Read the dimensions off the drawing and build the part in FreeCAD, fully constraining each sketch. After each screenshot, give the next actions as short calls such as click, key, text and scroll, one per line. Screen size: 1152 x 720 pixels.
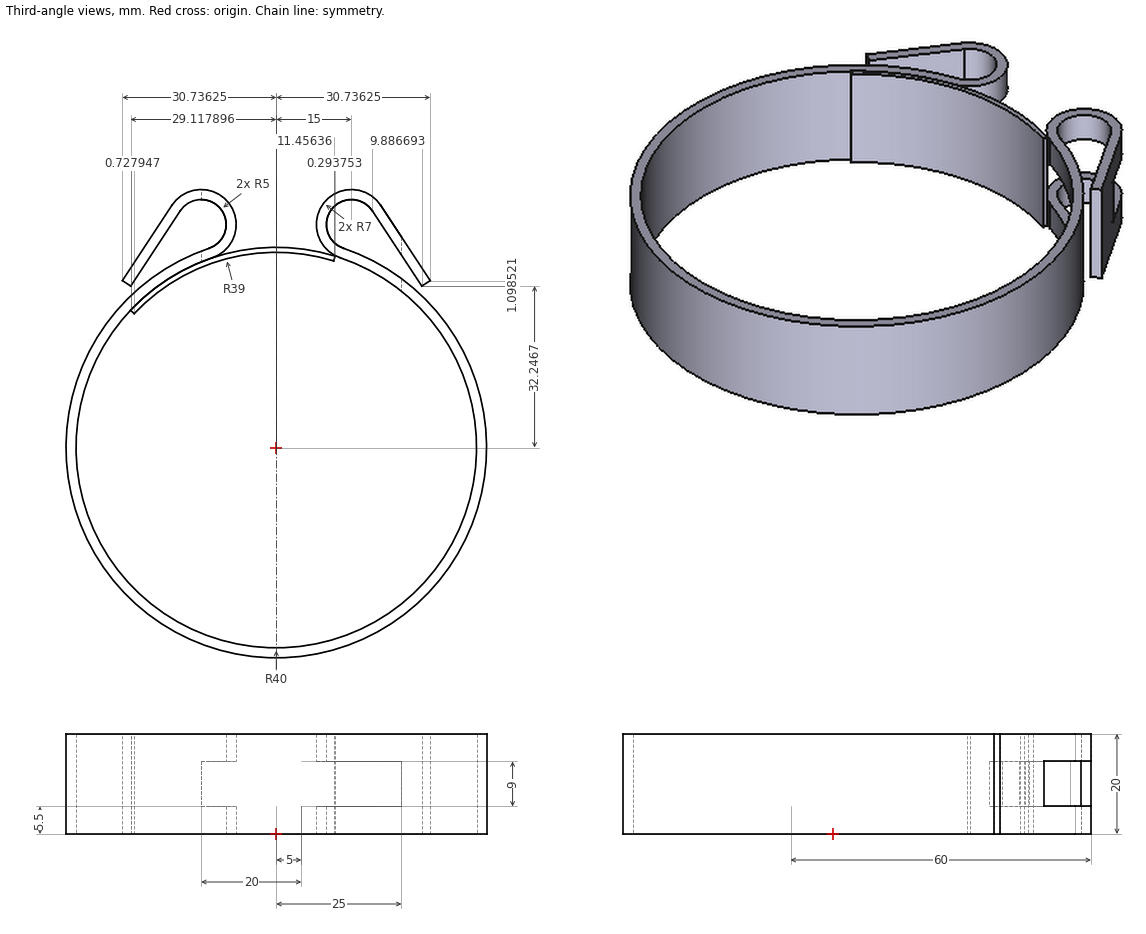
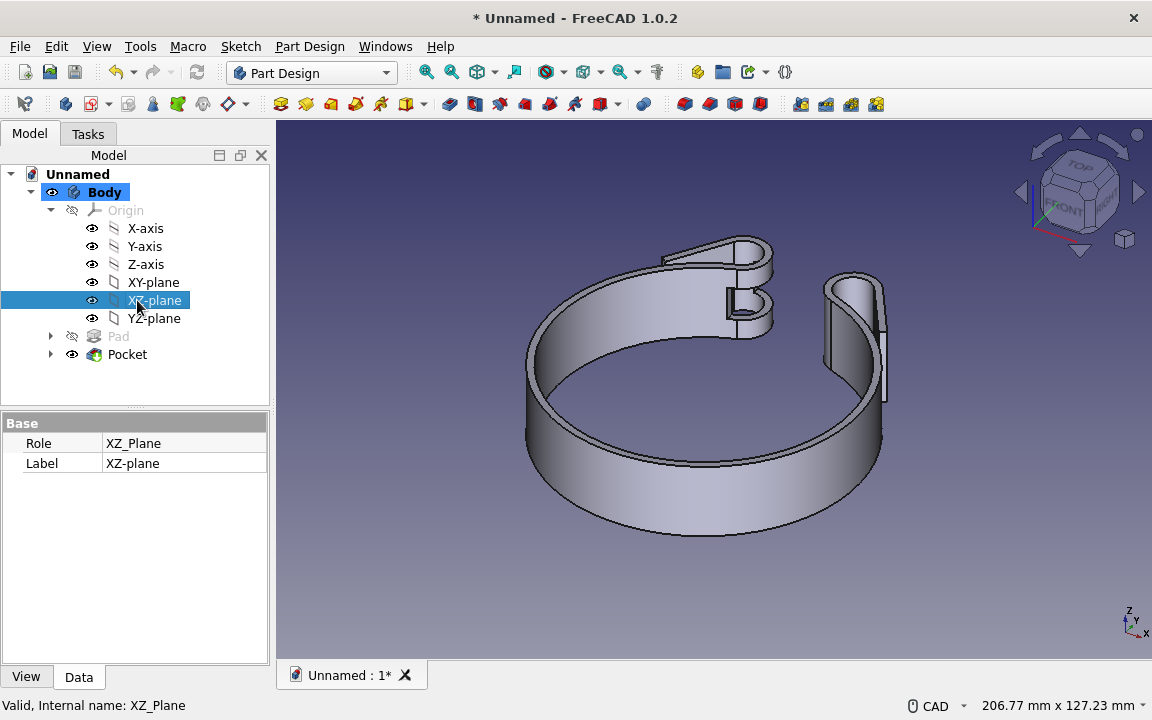
click(228, 104)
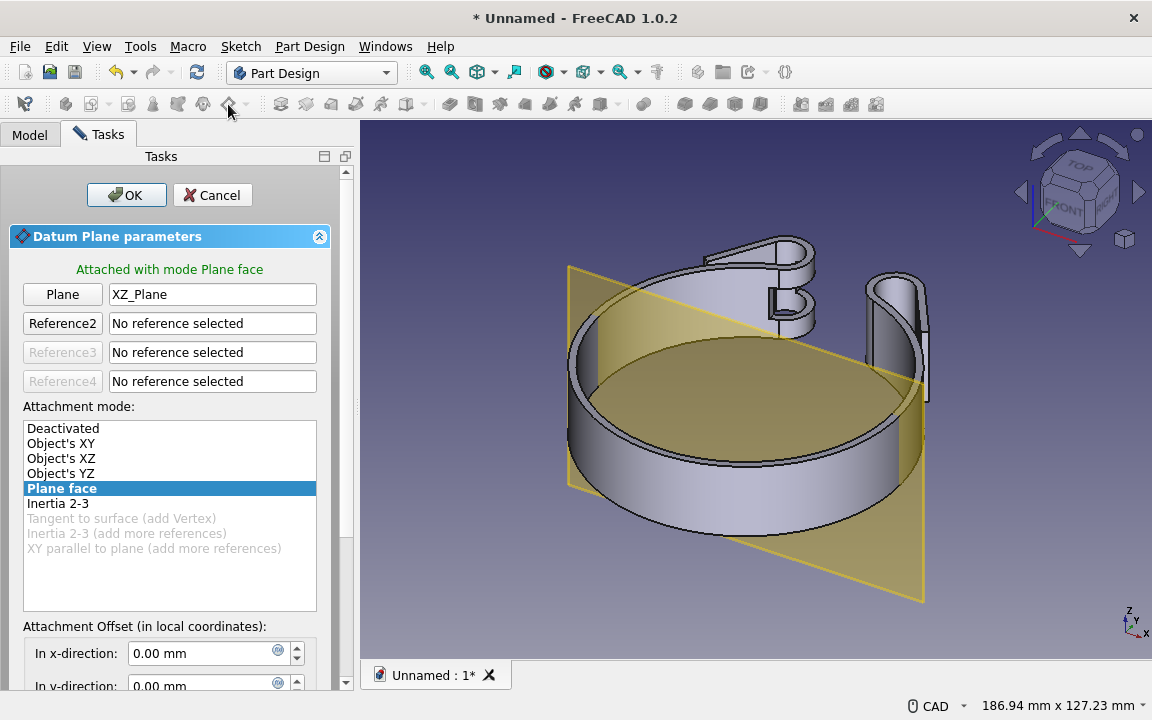
scroll(346, 428, down, 2)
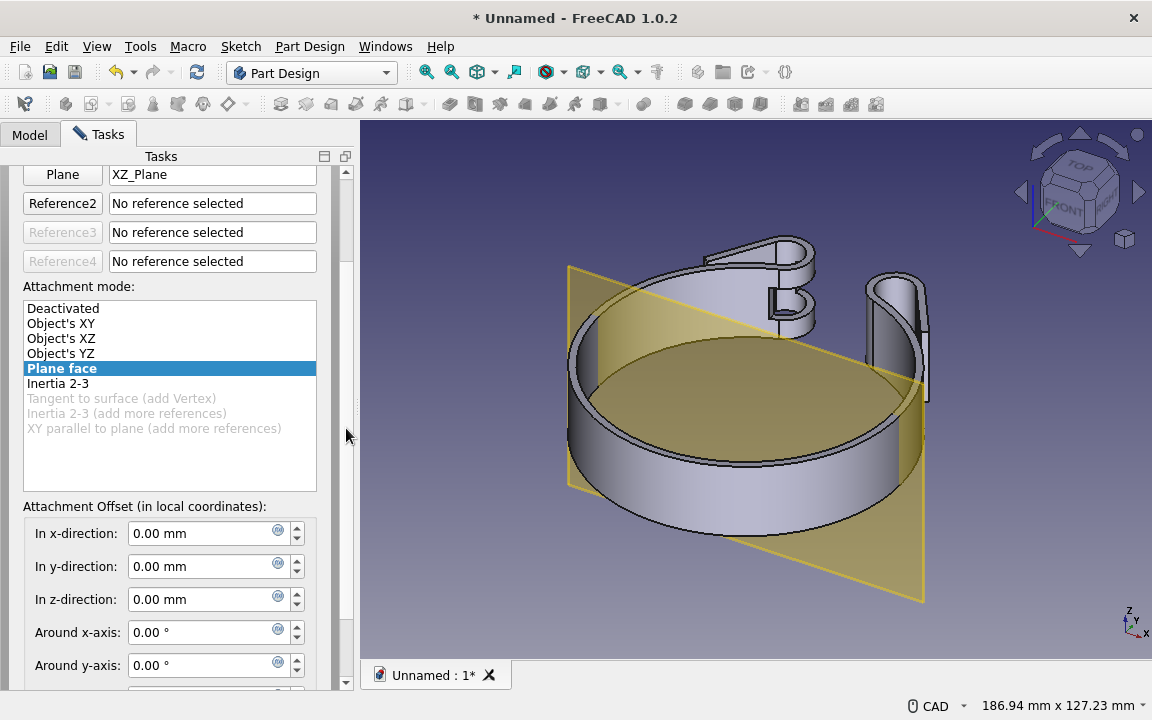
triple_click(210, 600)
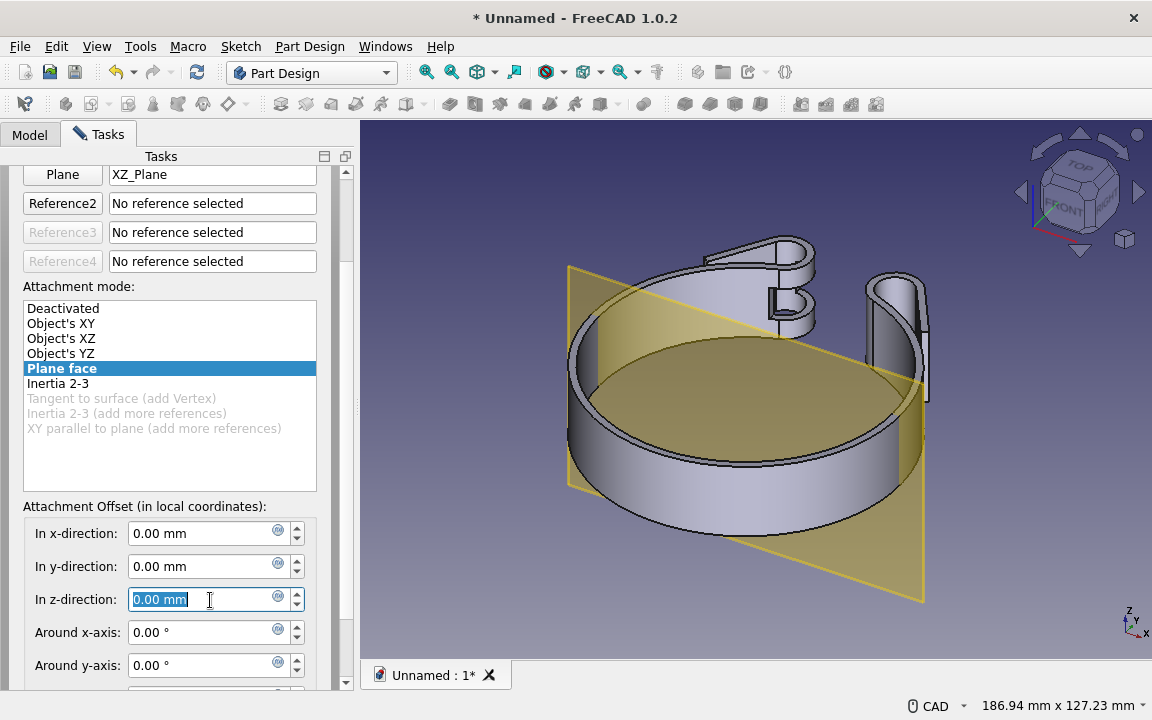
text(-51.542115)
key(Tab)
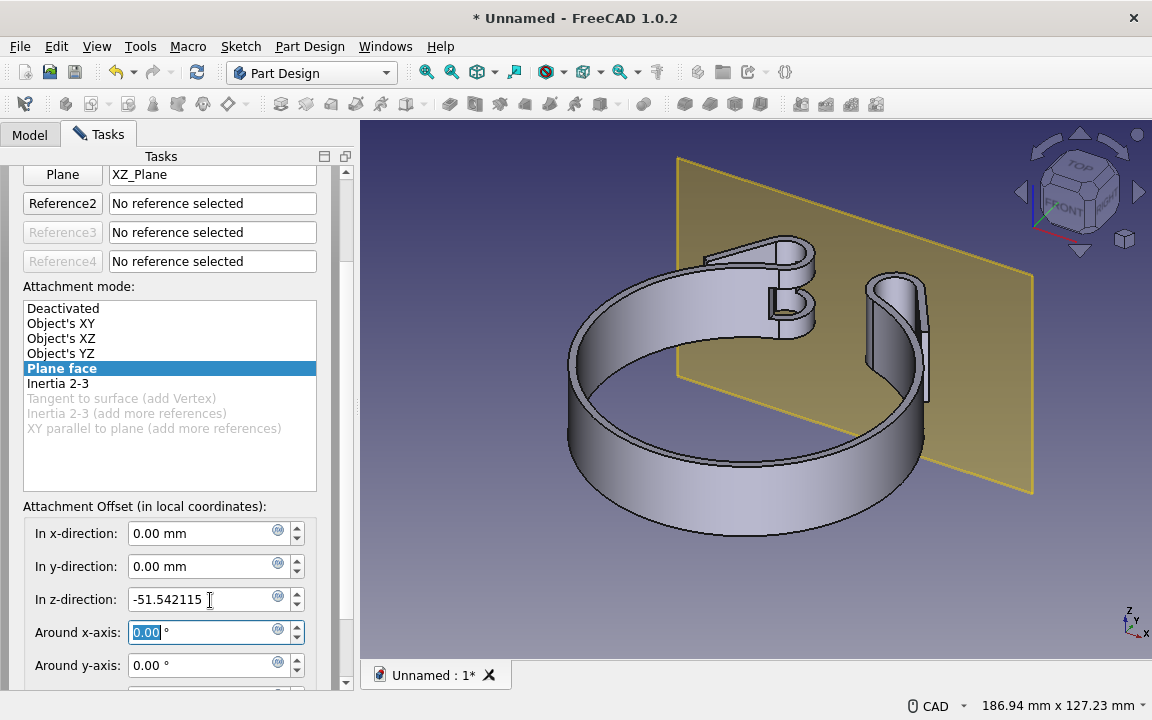
scroll(346, 428, up, 3)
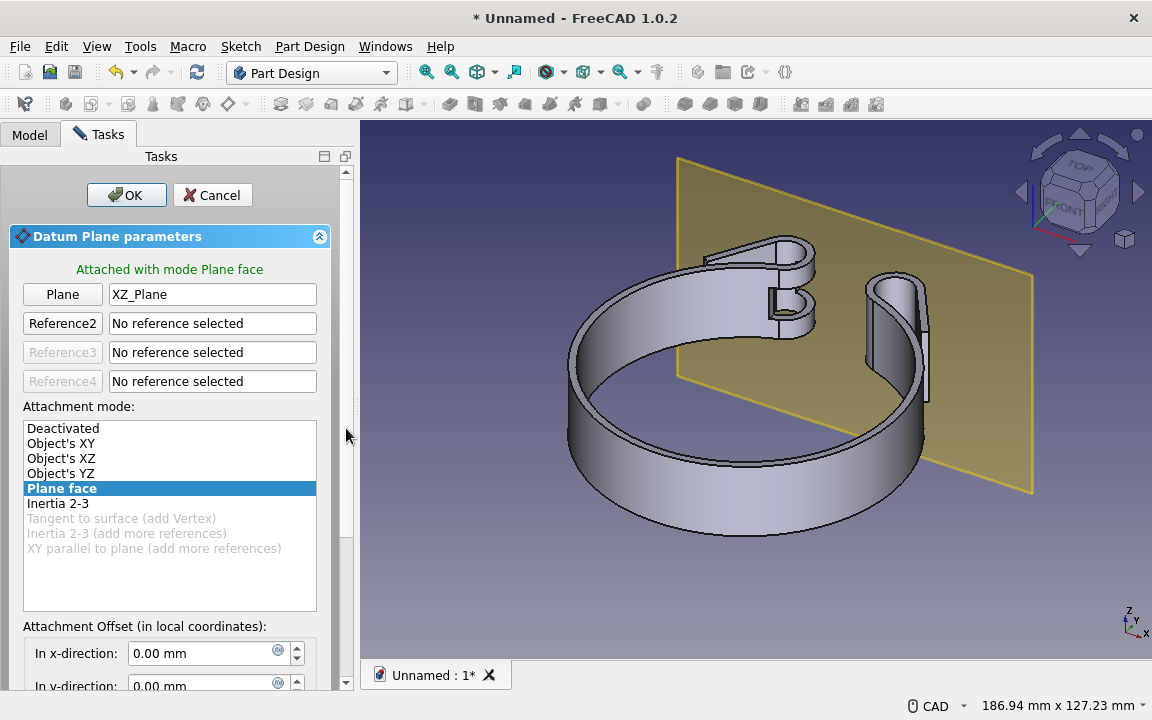
click(127, 195)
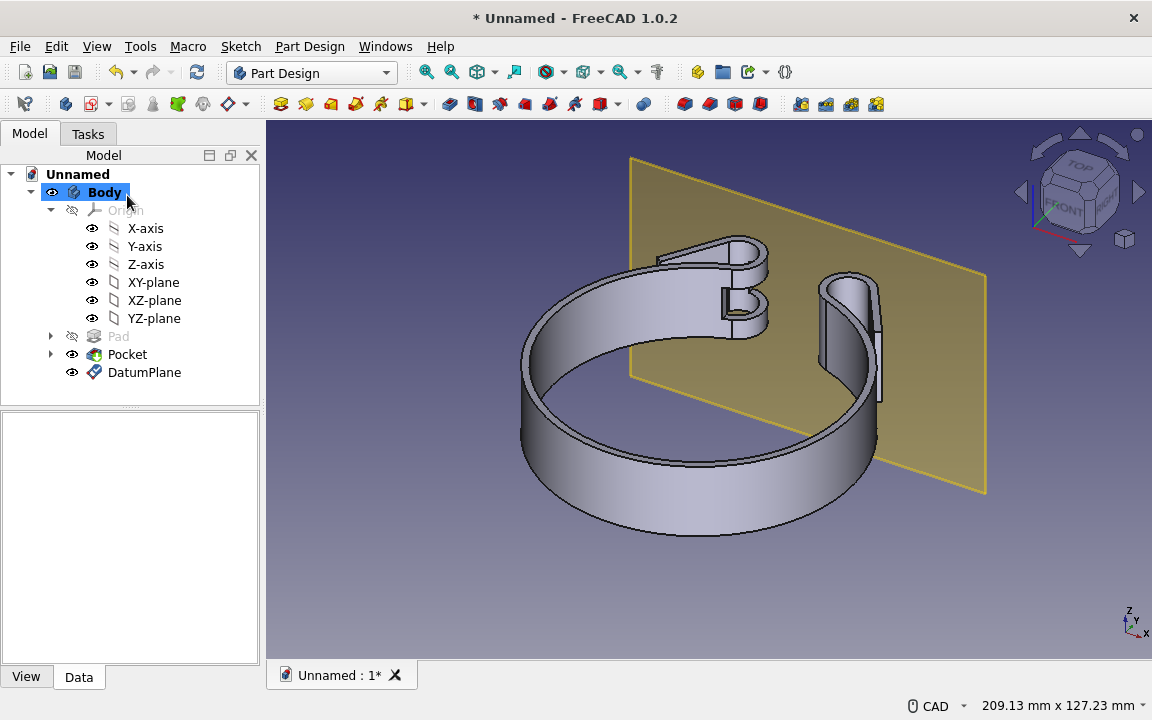
click(117, 372)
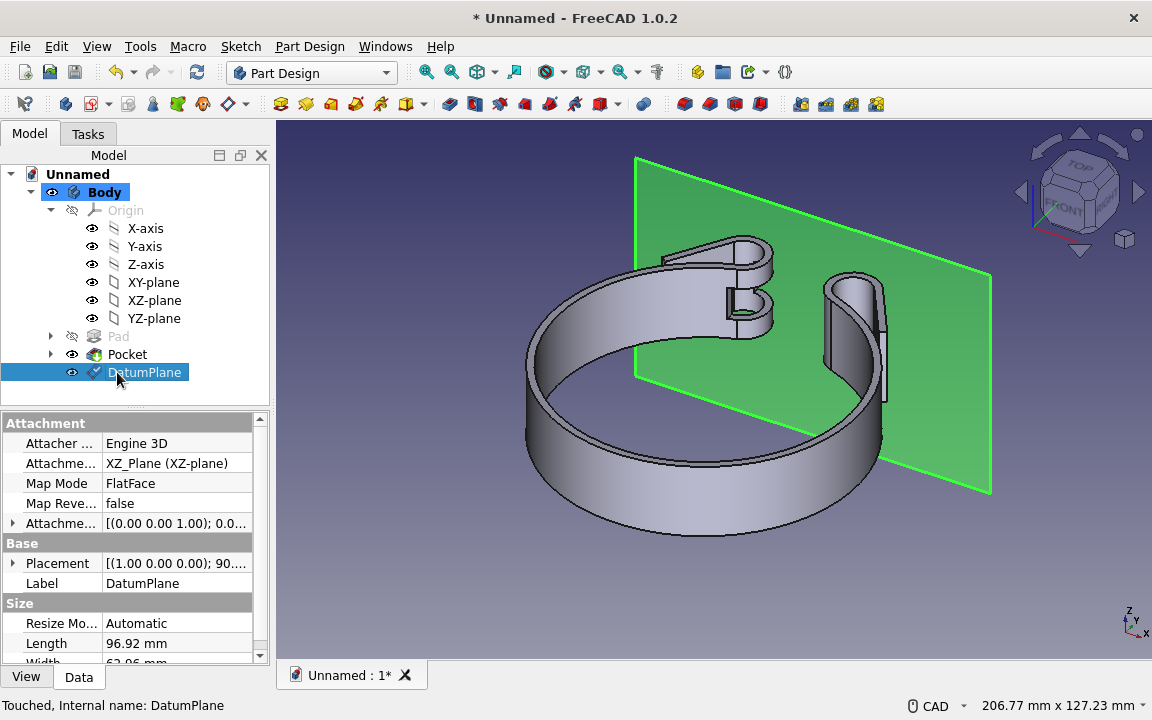
click(90, 104)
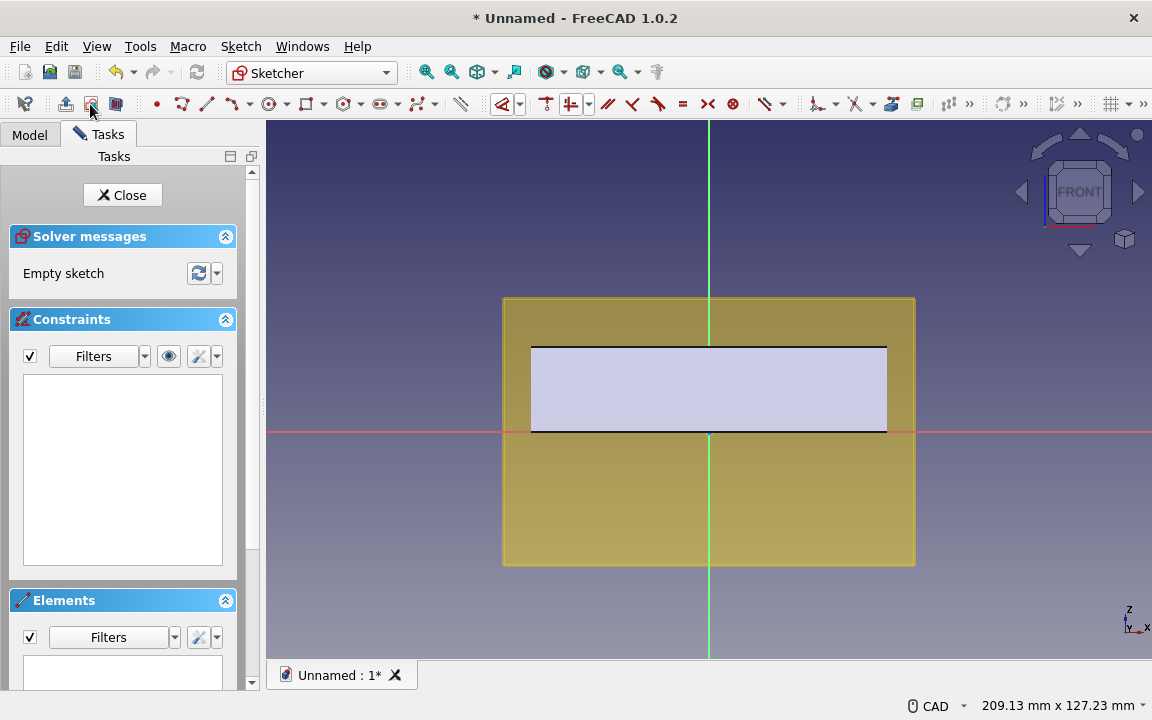
key(q)
key(s)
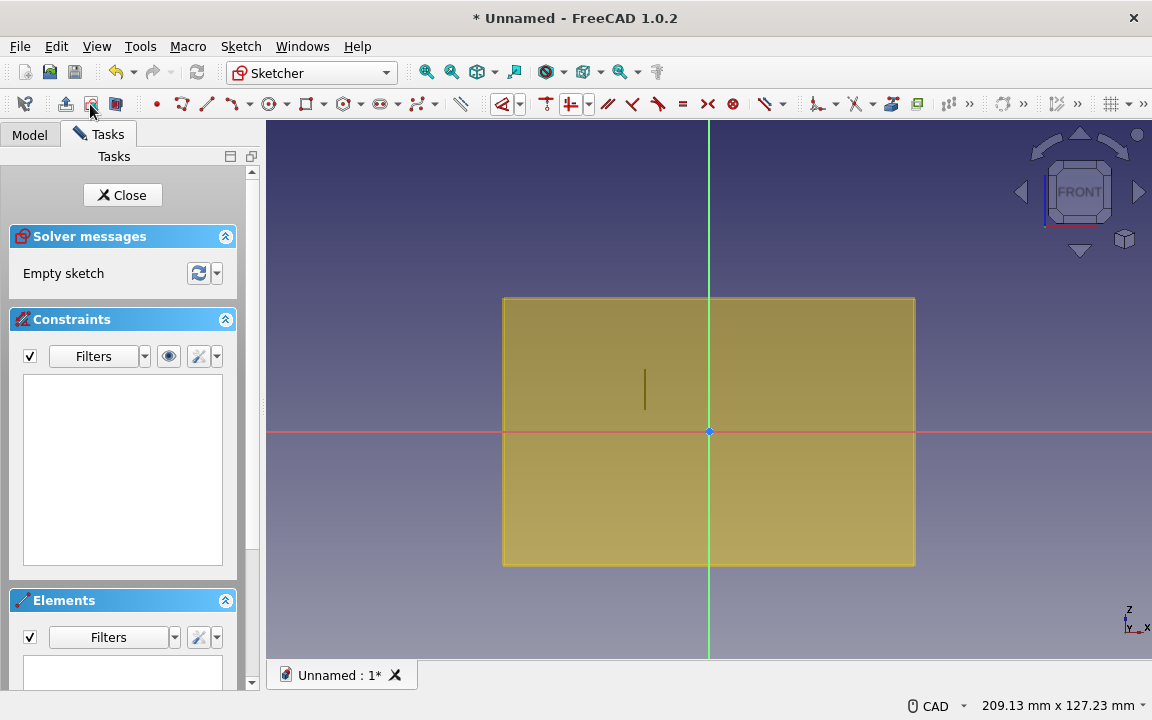
scroll(793, 404, up, 8)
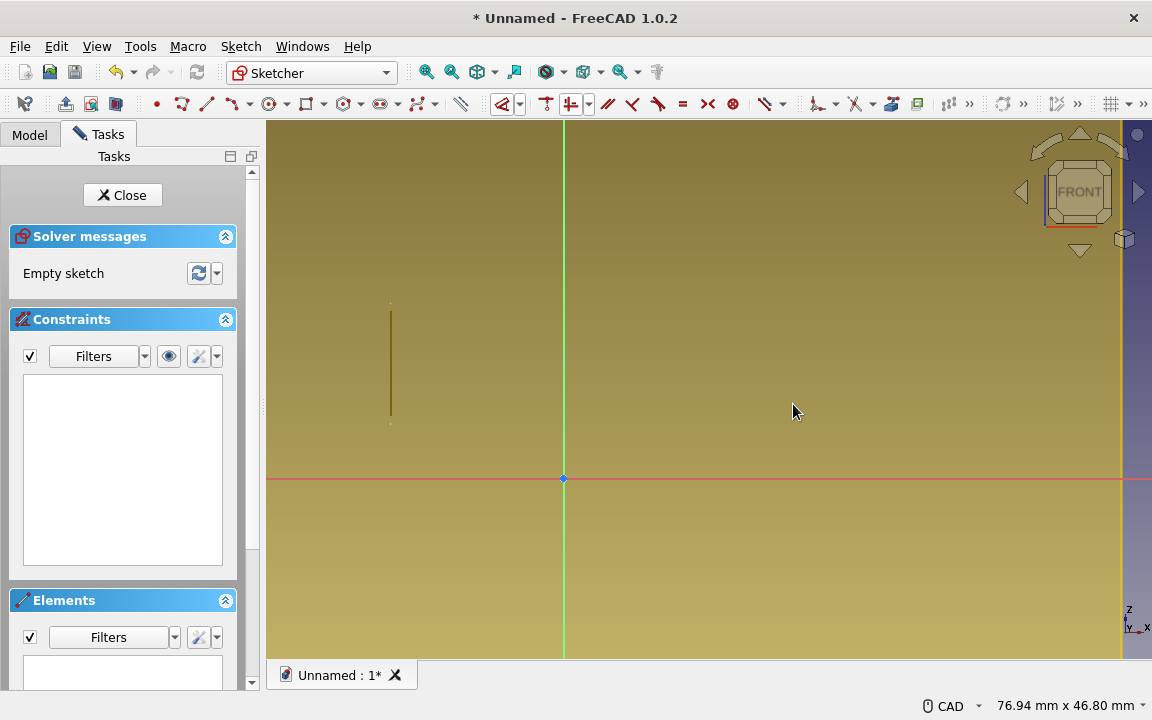
key(g)
key(r)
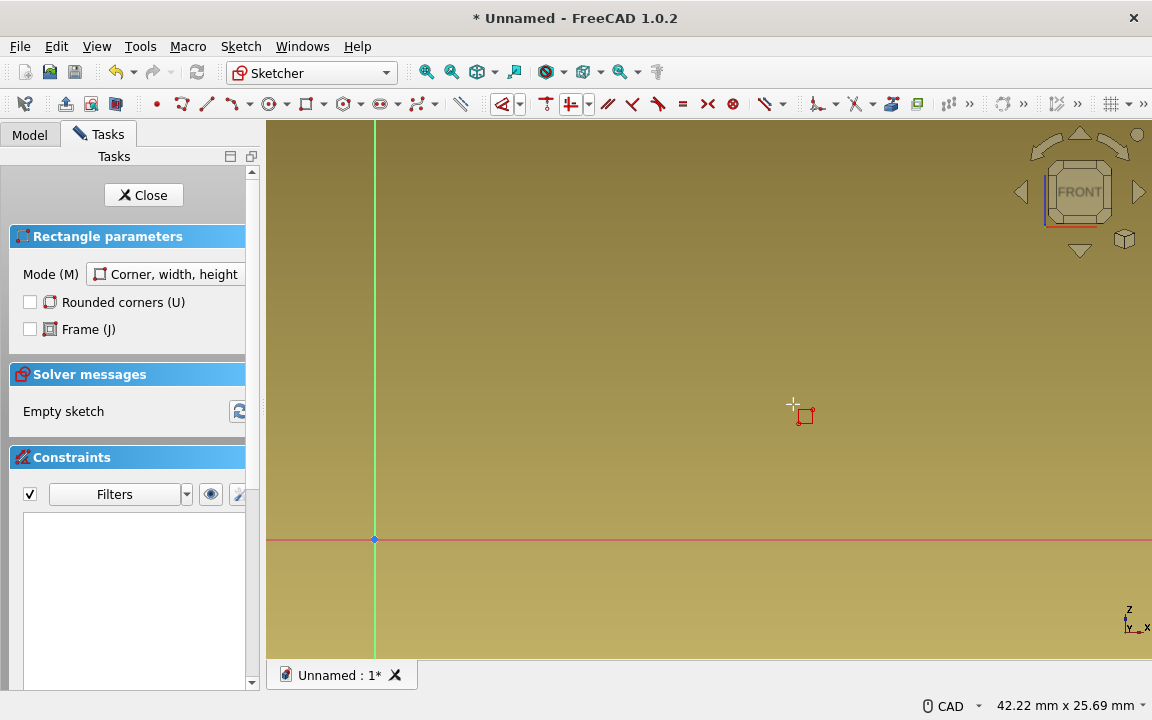
click(375, 236)
move(899, 425)